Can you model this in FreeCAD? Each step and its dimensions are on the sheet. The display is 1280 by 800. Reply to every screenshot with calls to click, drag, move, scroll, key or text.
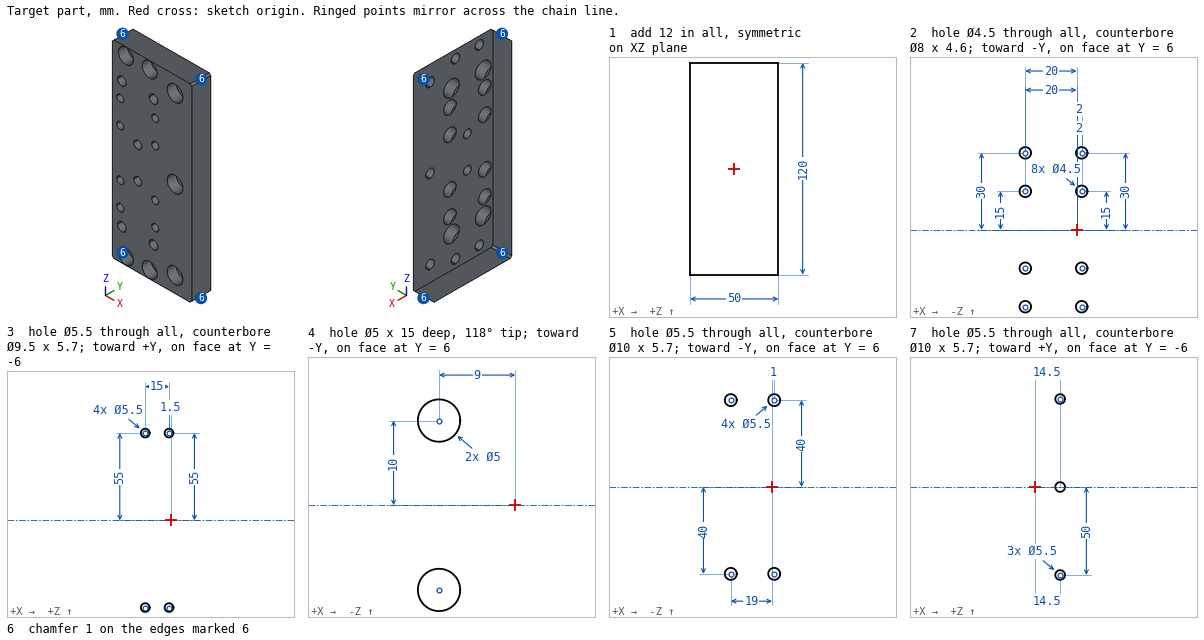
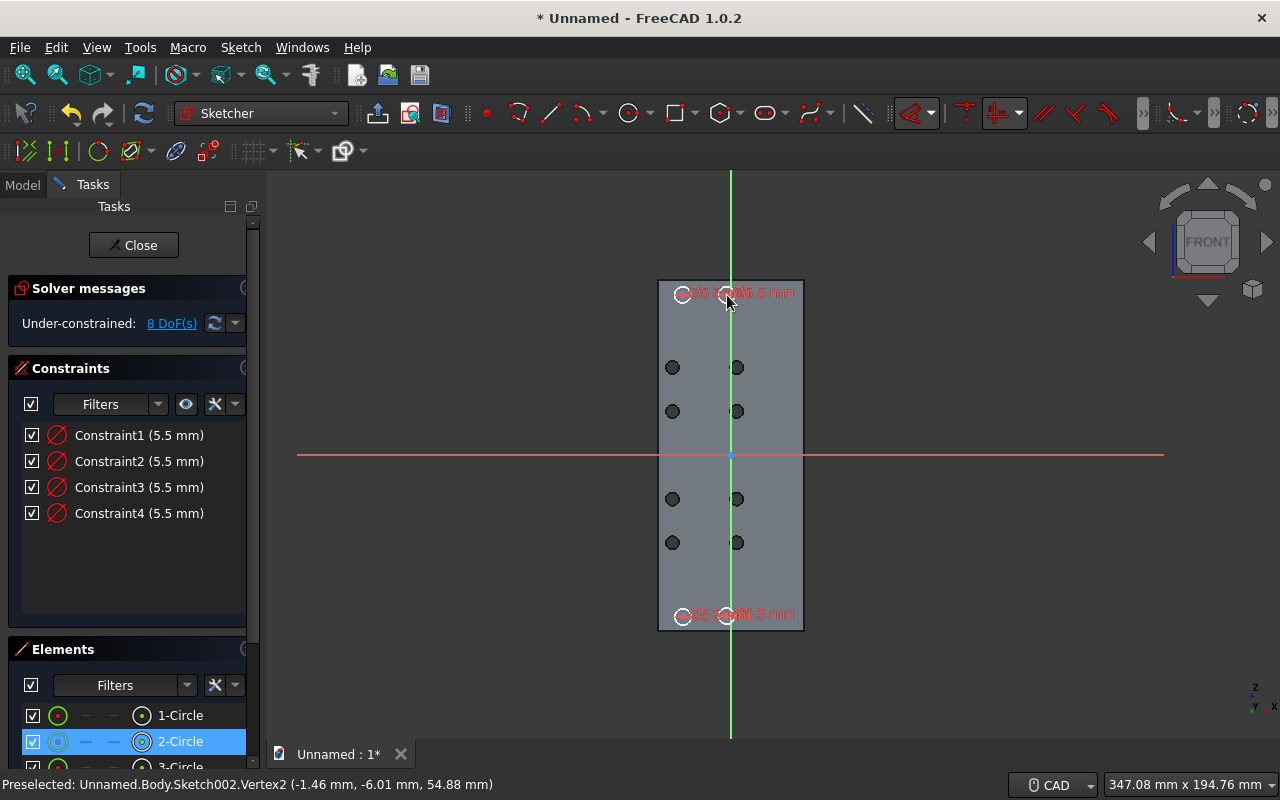
click(727, 616)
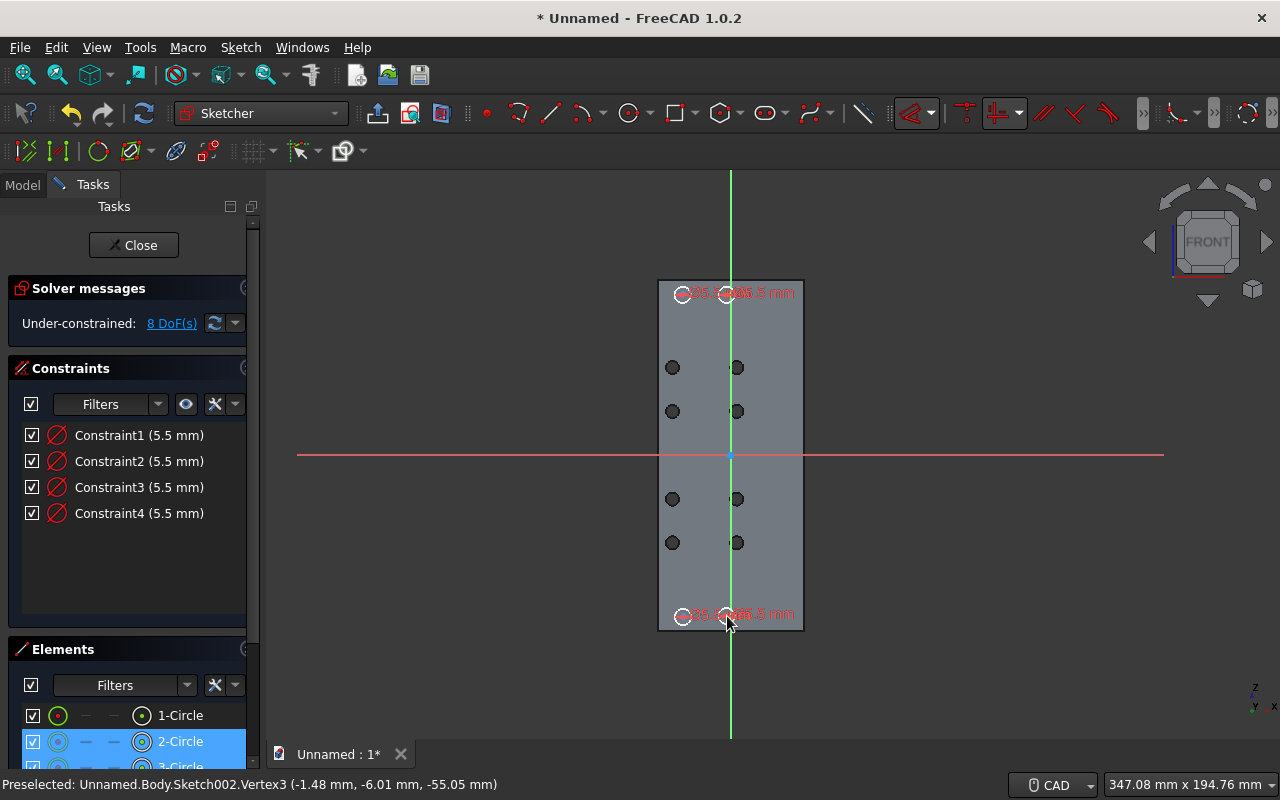
click(353, 455)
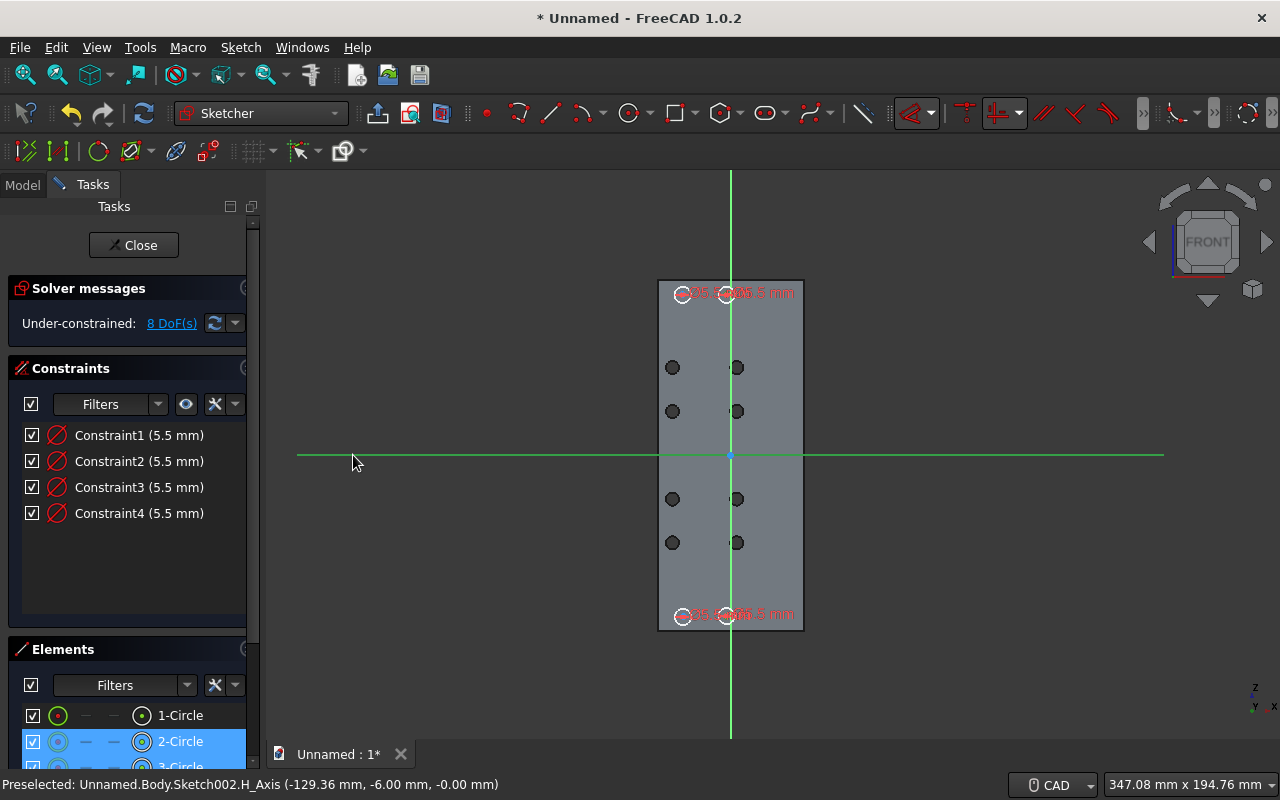
key(s)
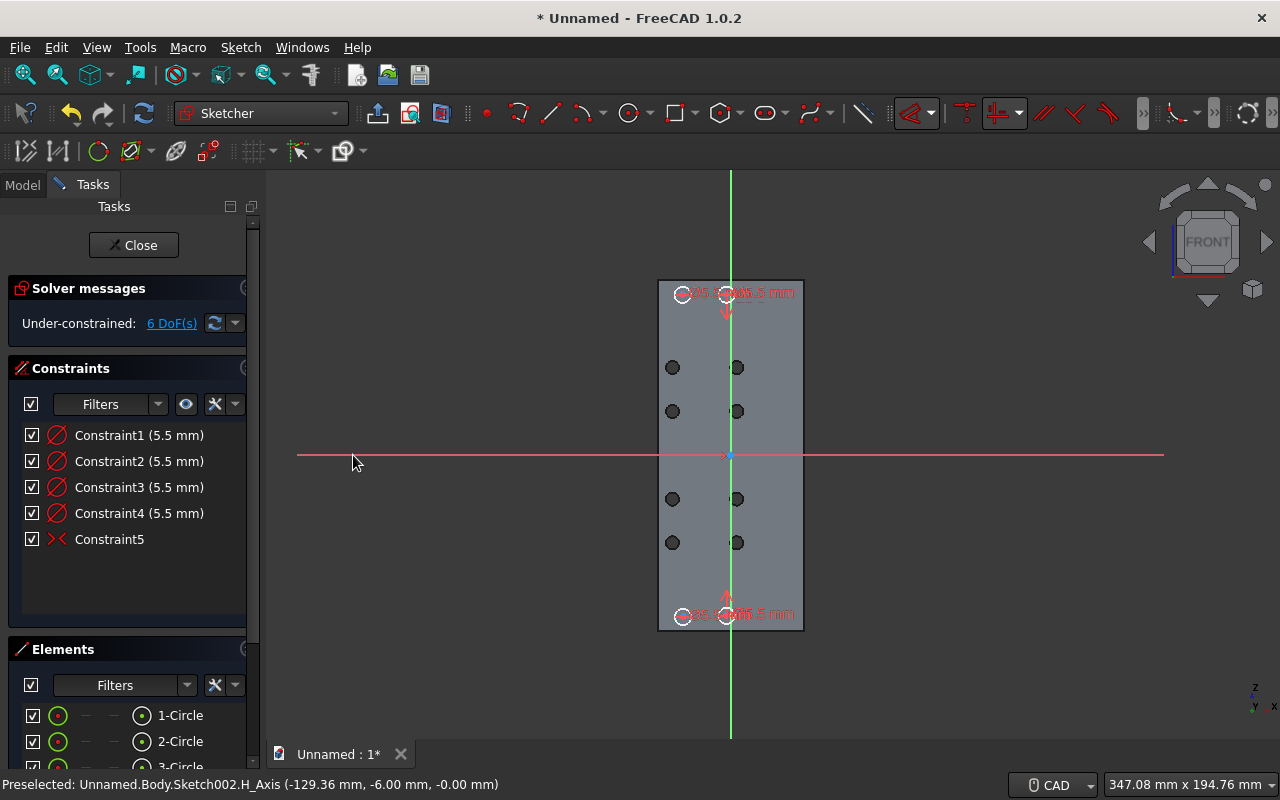
click(683, 295)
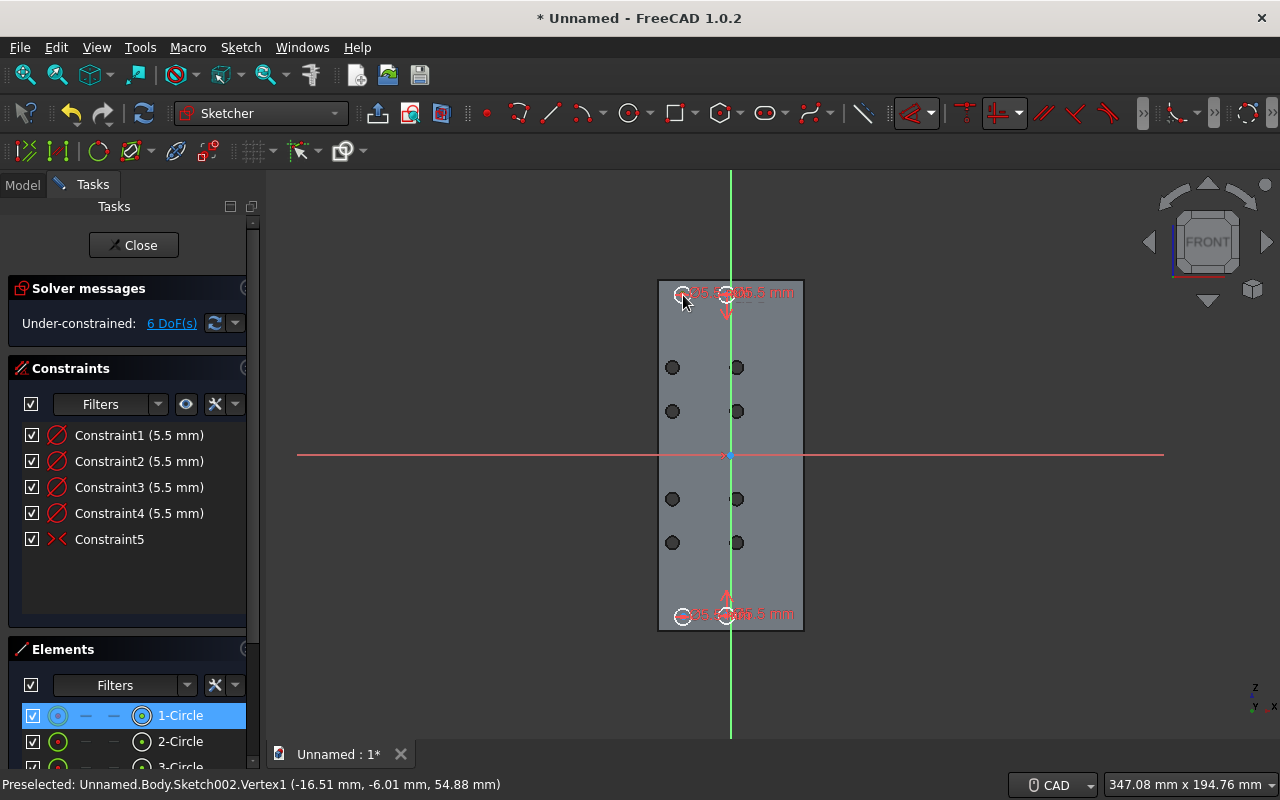
click(683, 617)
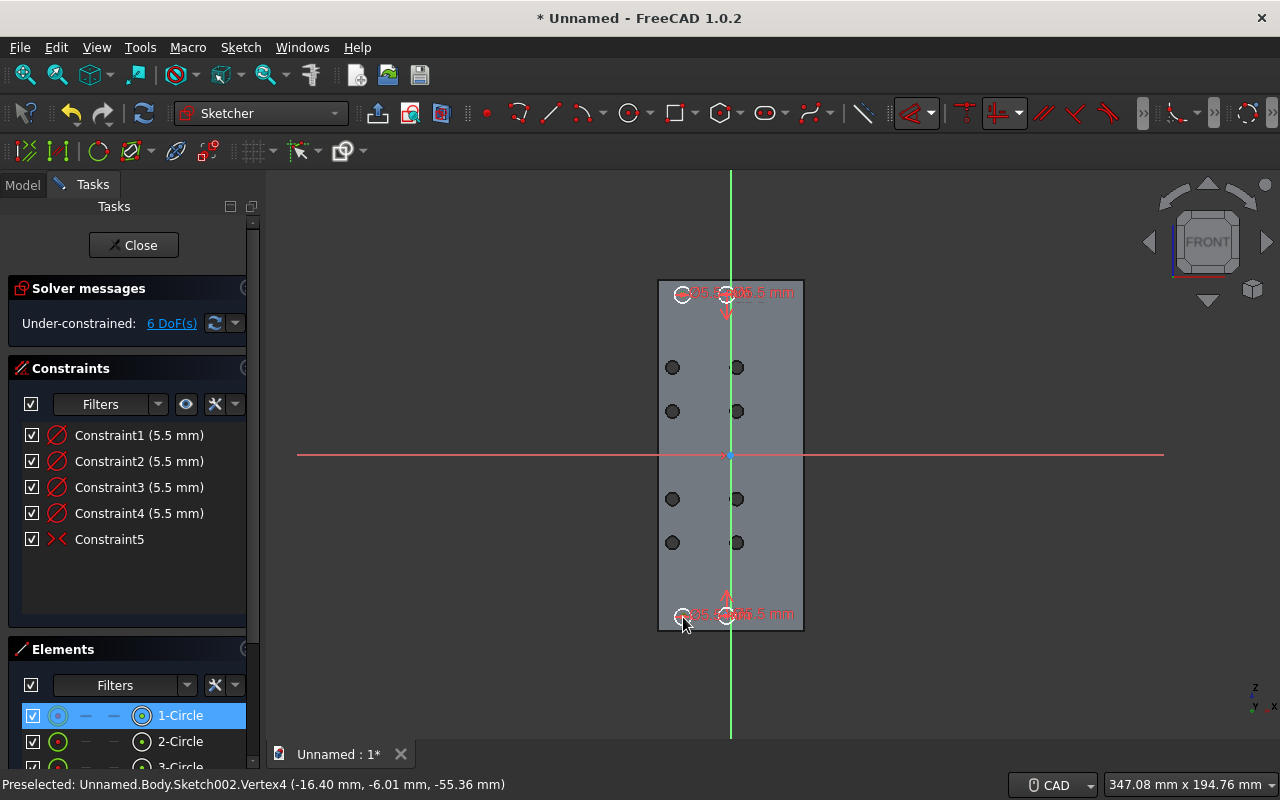
click(353, 455)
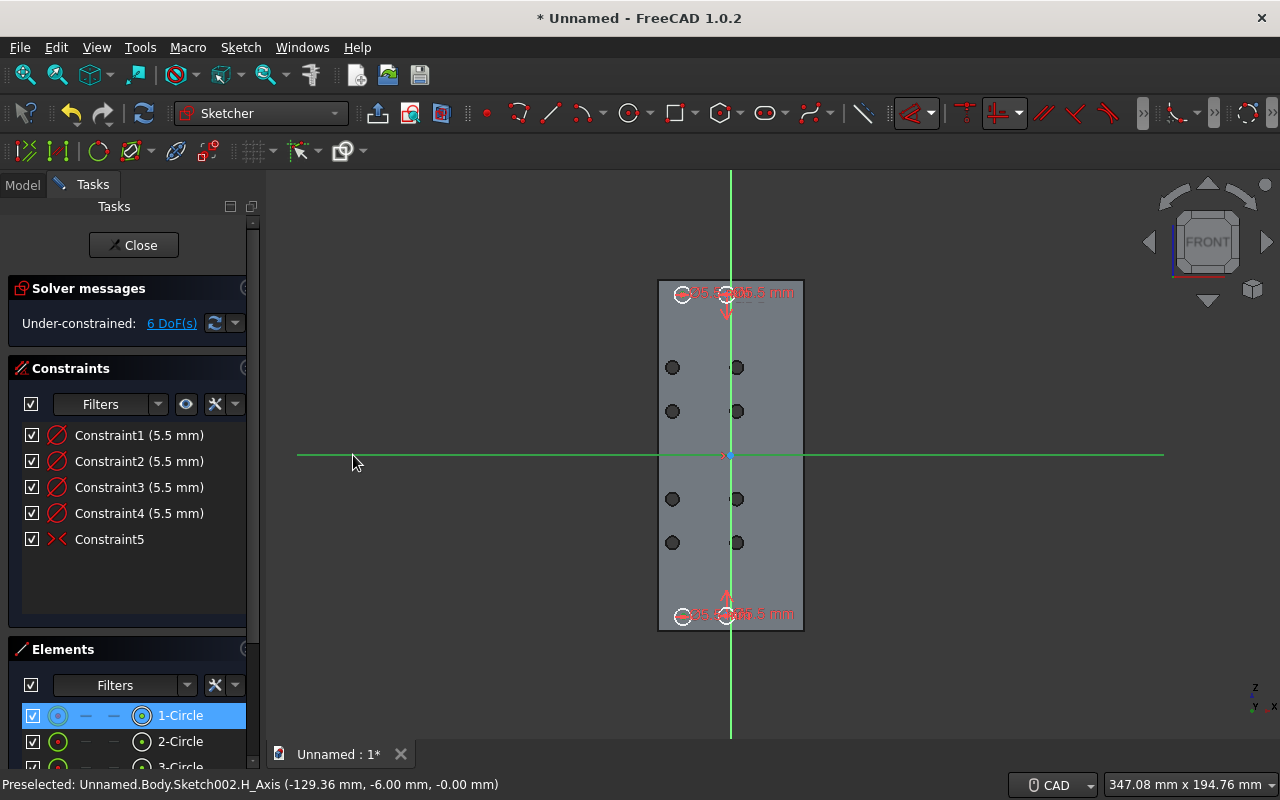
key(s)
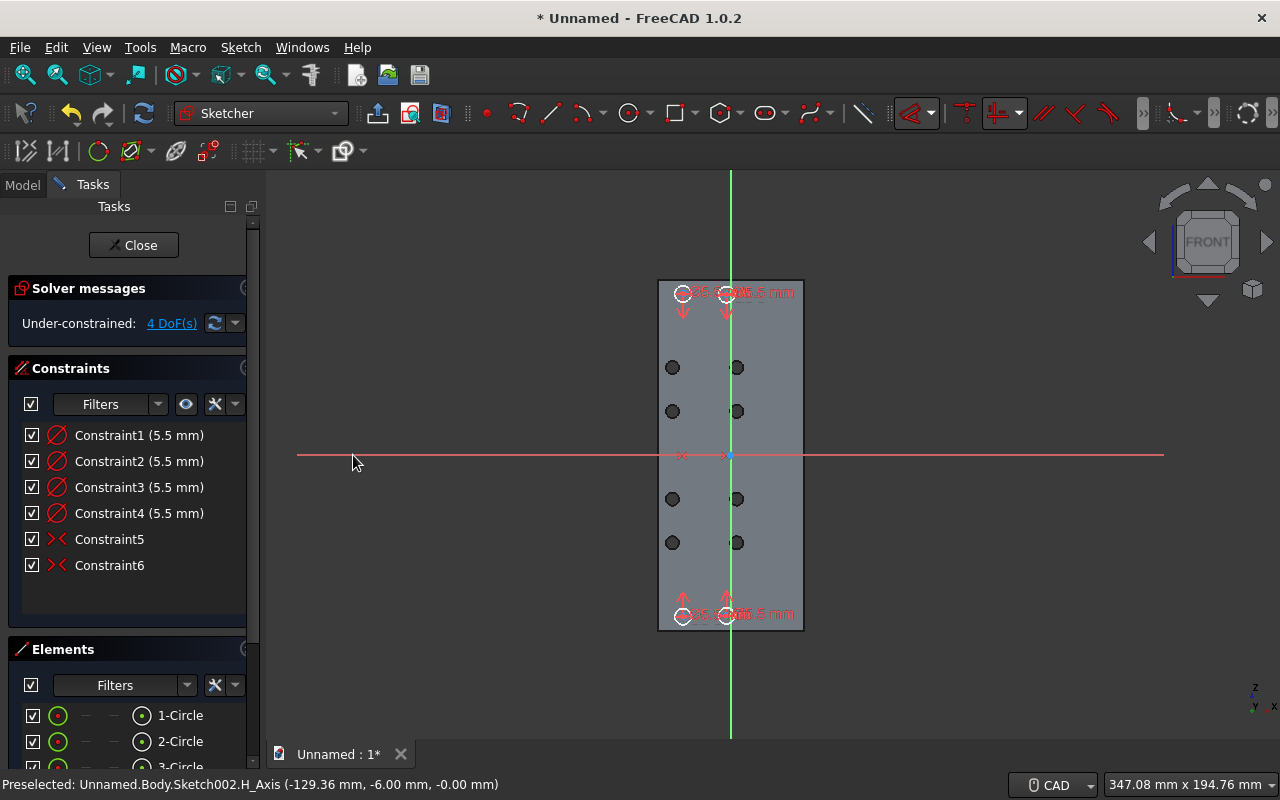
click(683, 294)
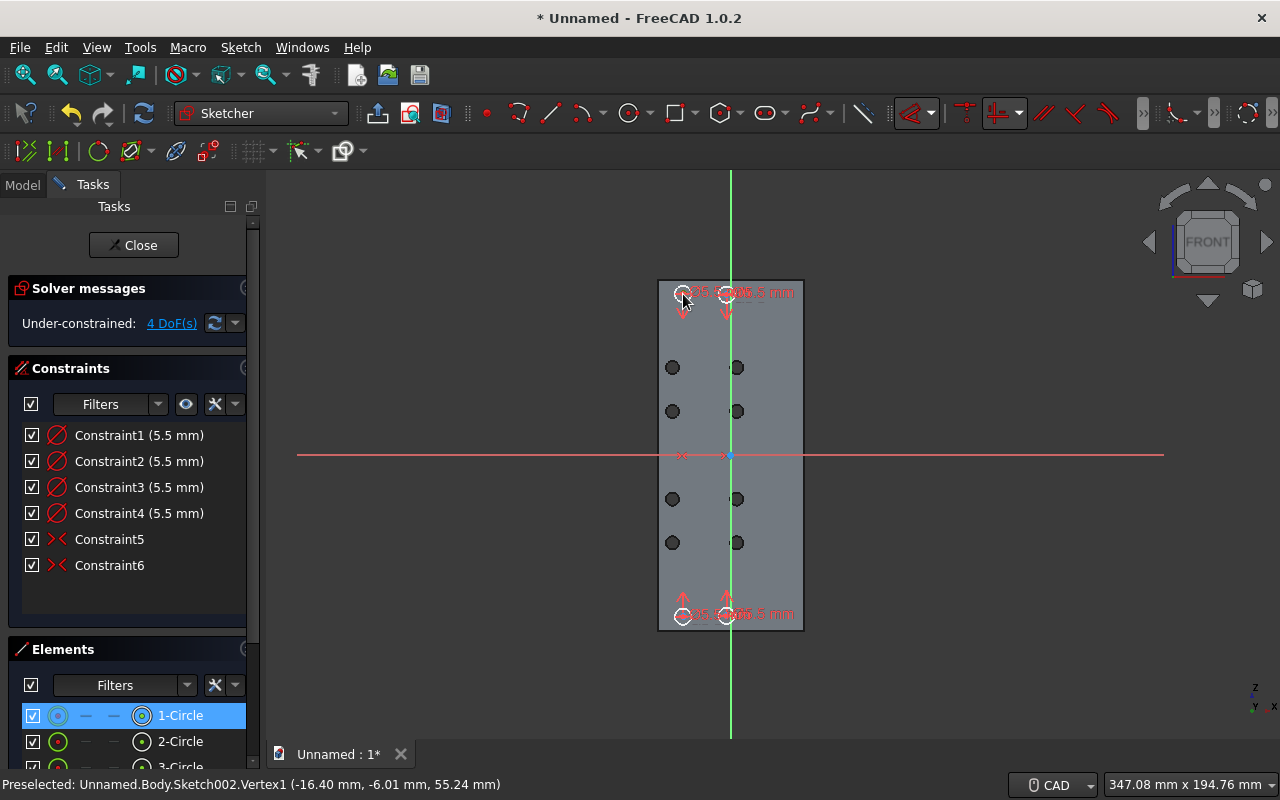
click(934, 114)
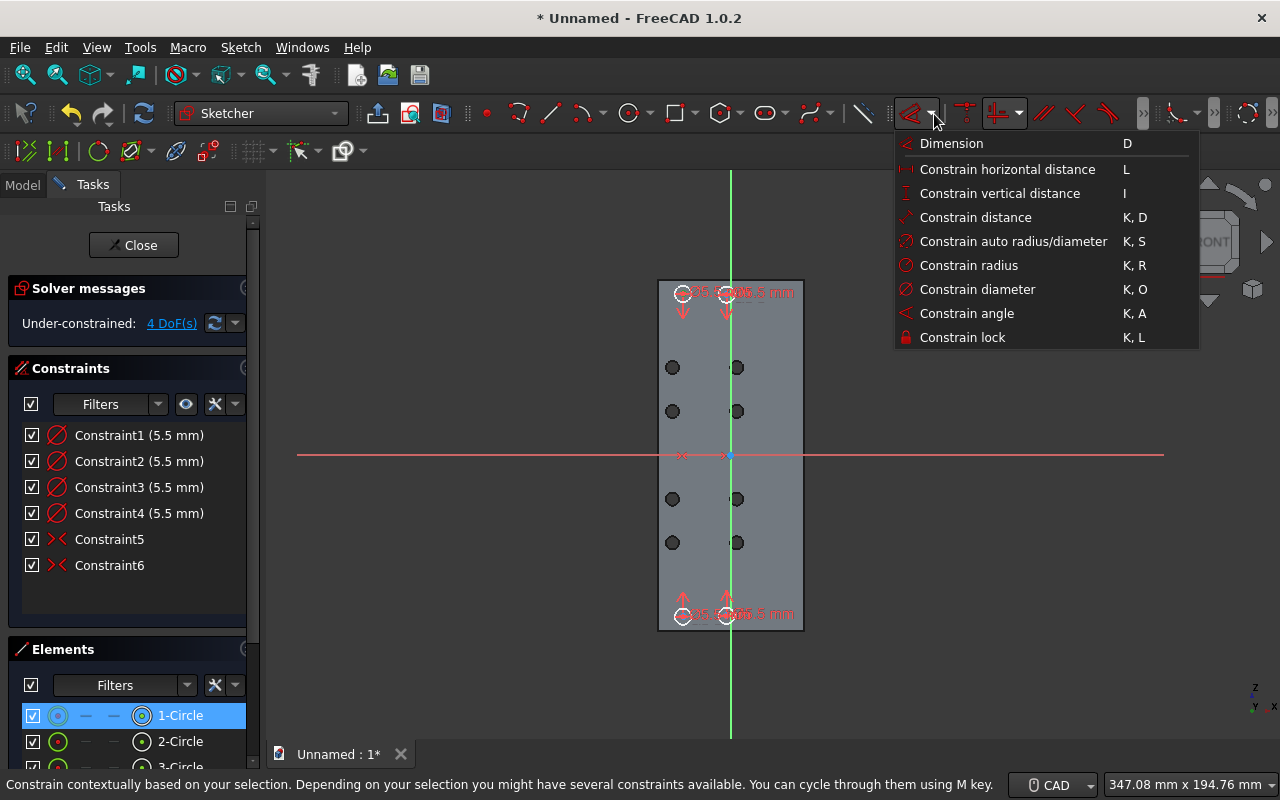
click(1047, 193)